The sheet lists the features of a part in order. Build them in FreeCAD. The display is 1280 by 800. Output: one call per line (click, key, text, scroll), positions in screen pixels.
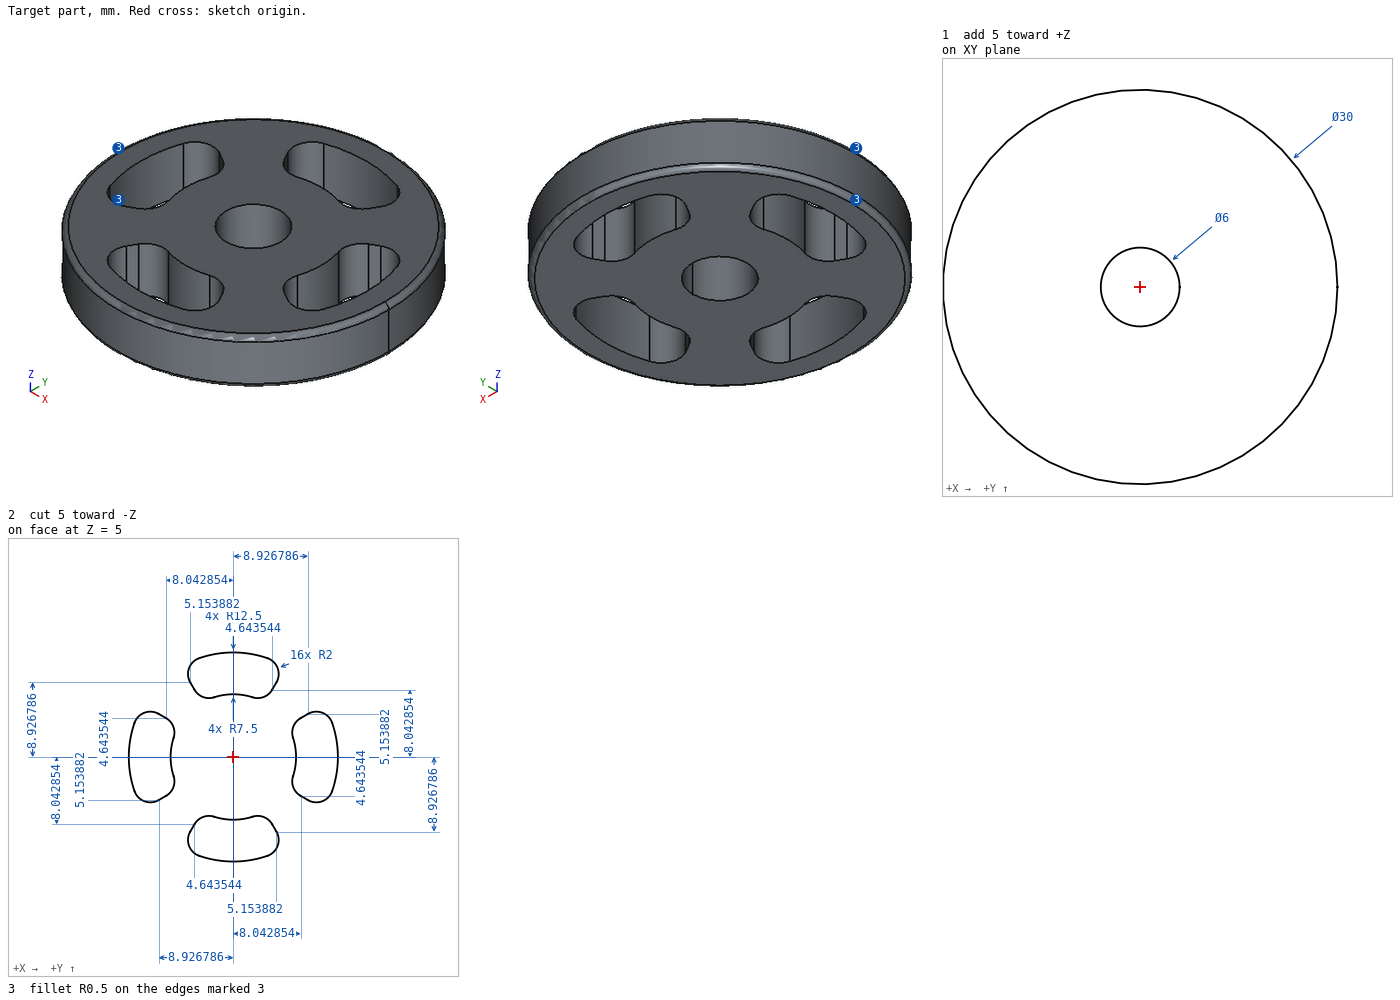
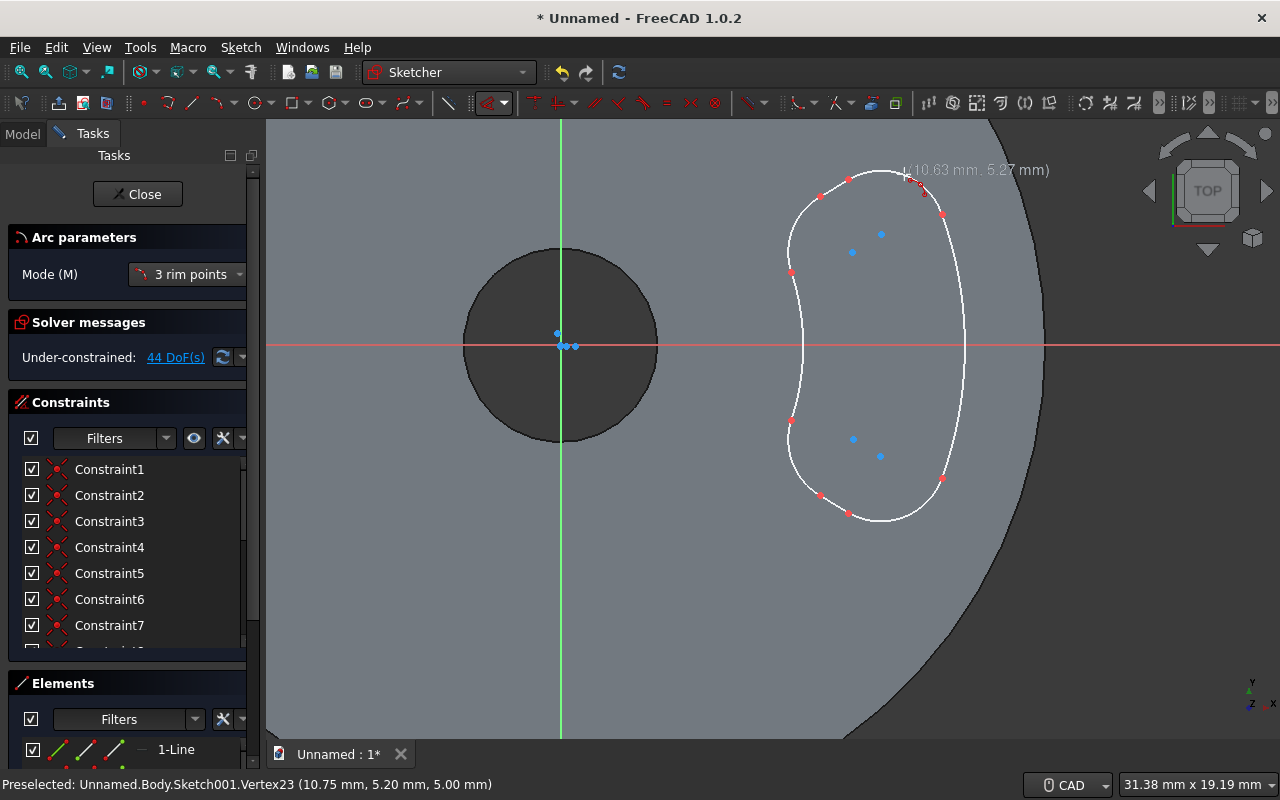
click(192, 104)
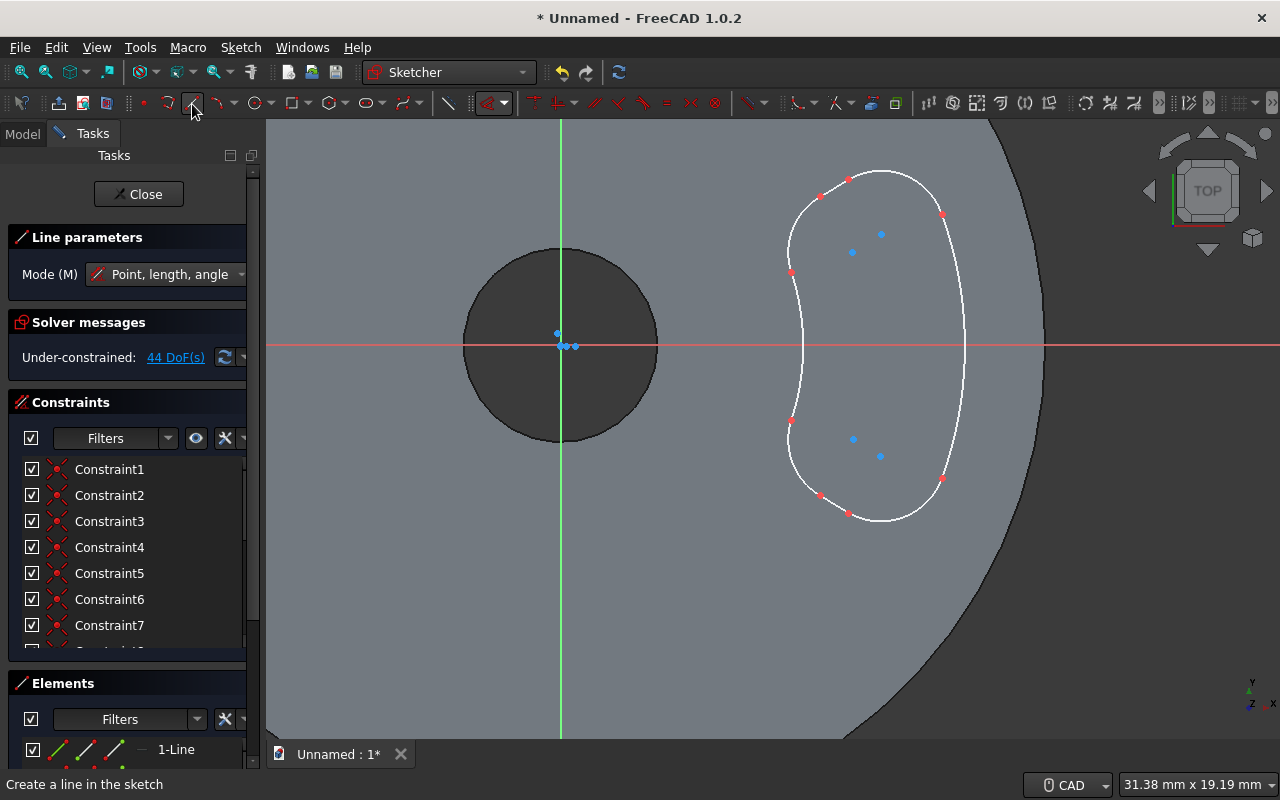
click(727, 634)
click(711, 605)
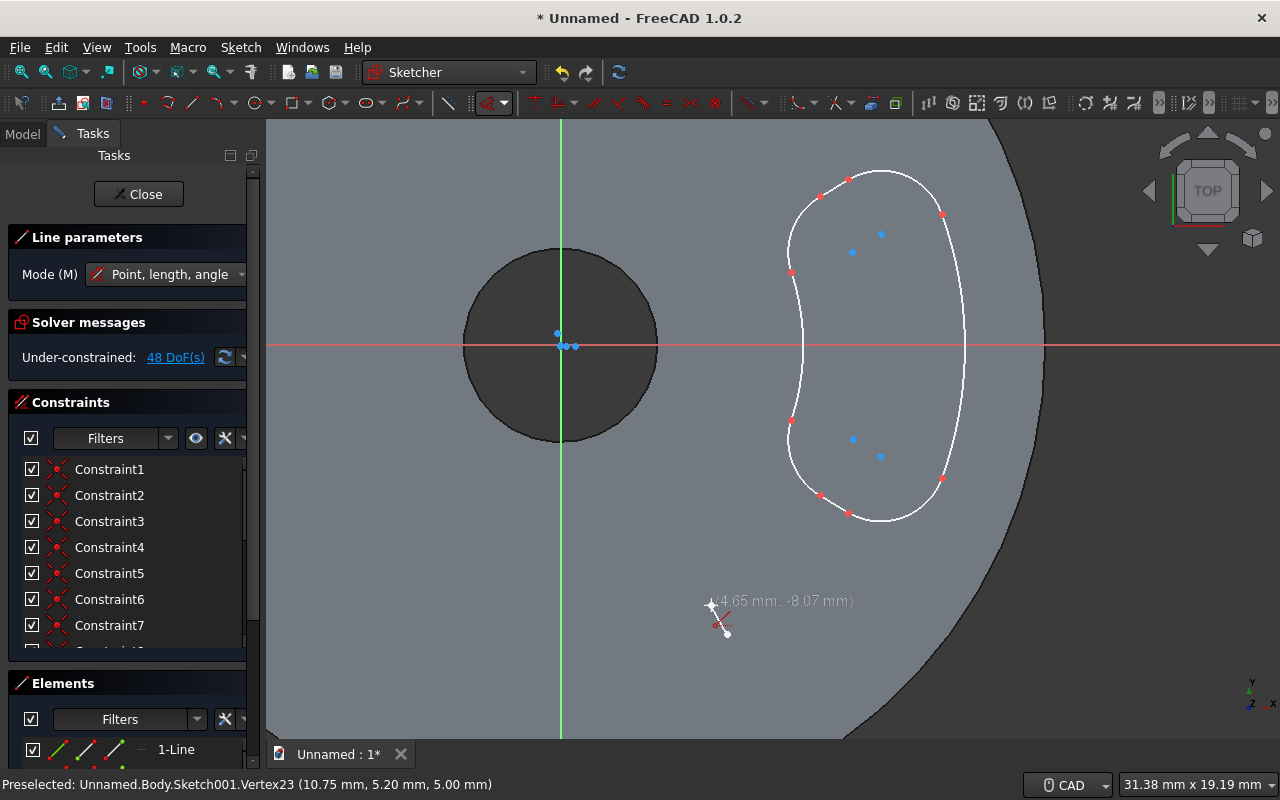
click(411, 605)
click(394, 634)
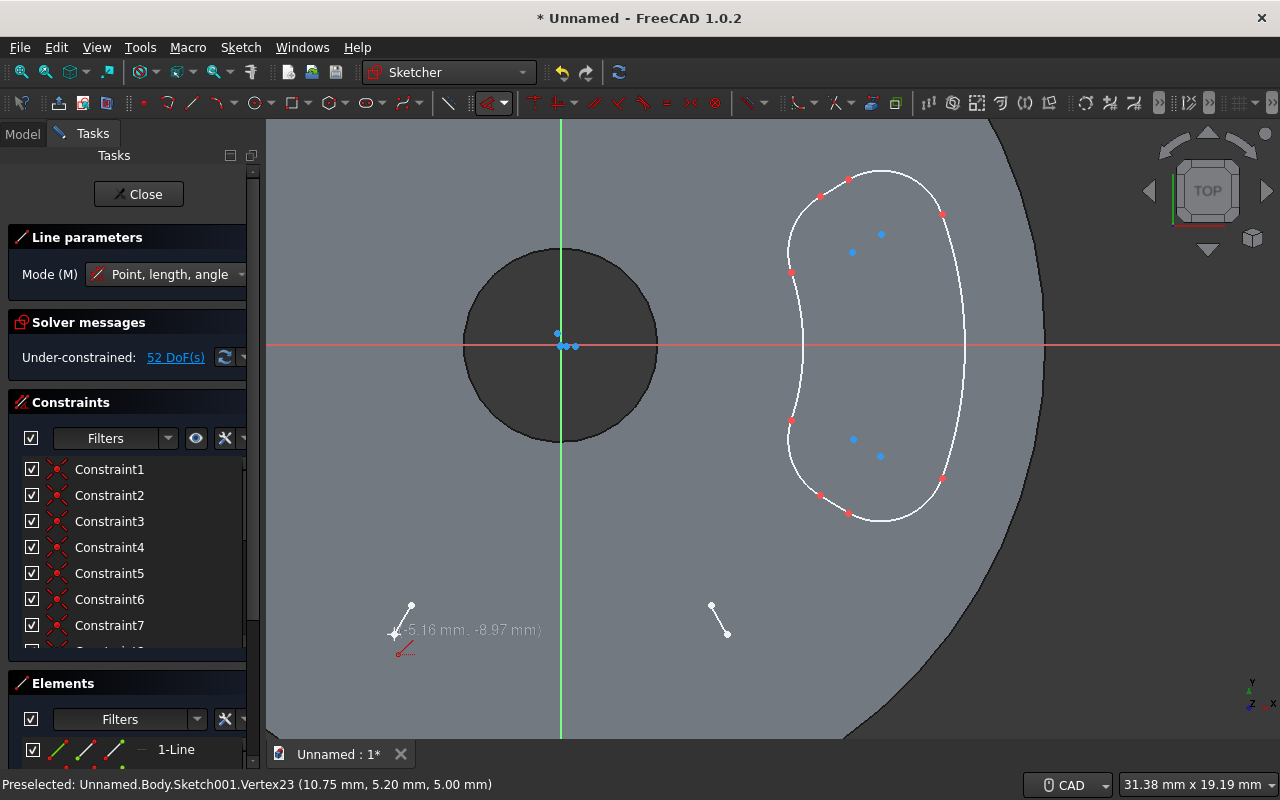
click(218, 104)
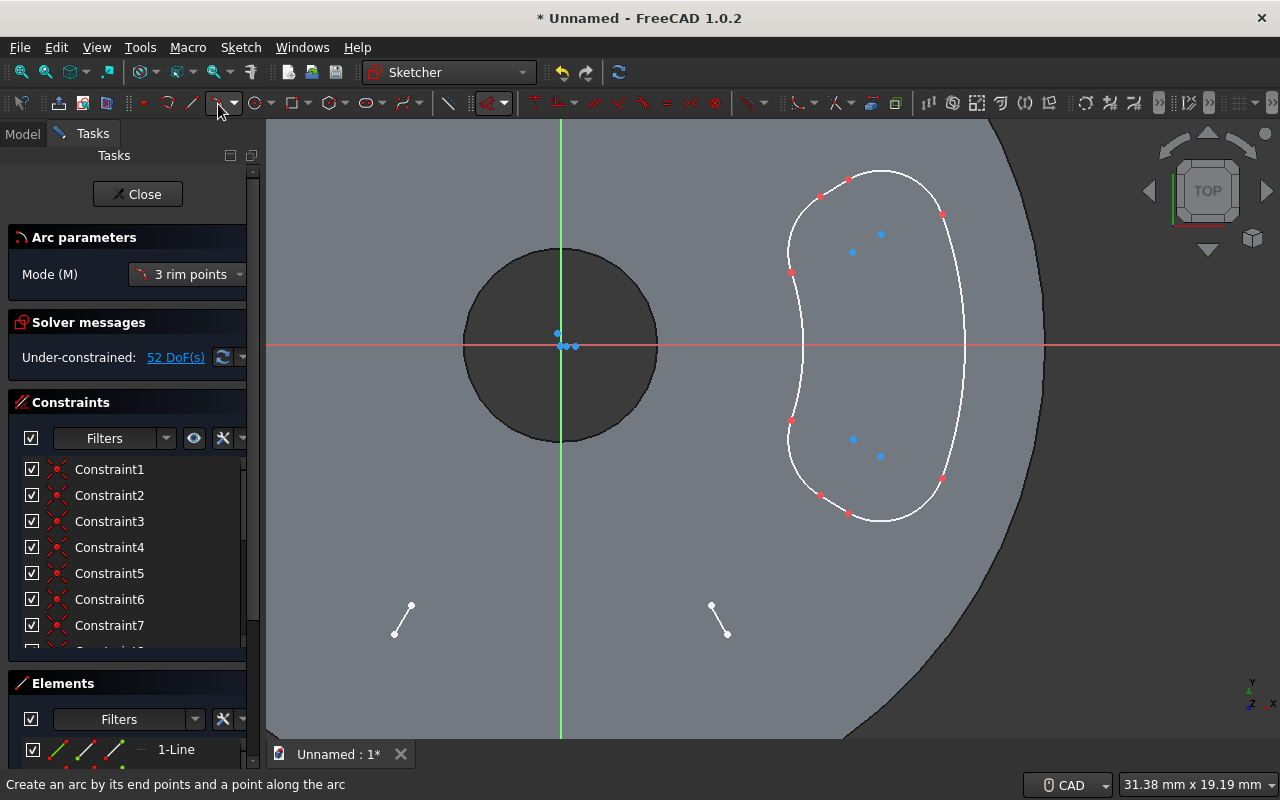
click(711, 606)
click(635, 576)
click(678, 577)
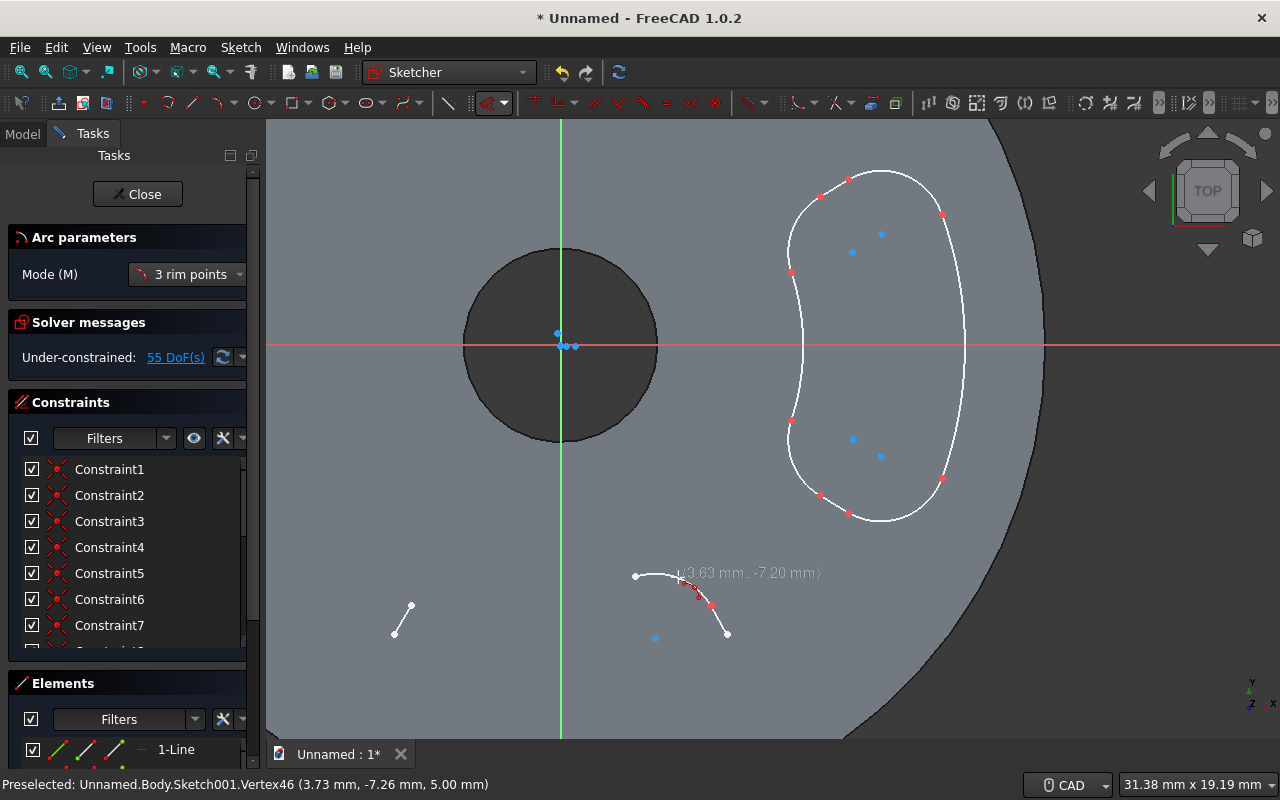
click(635, 577)
click(486, 576)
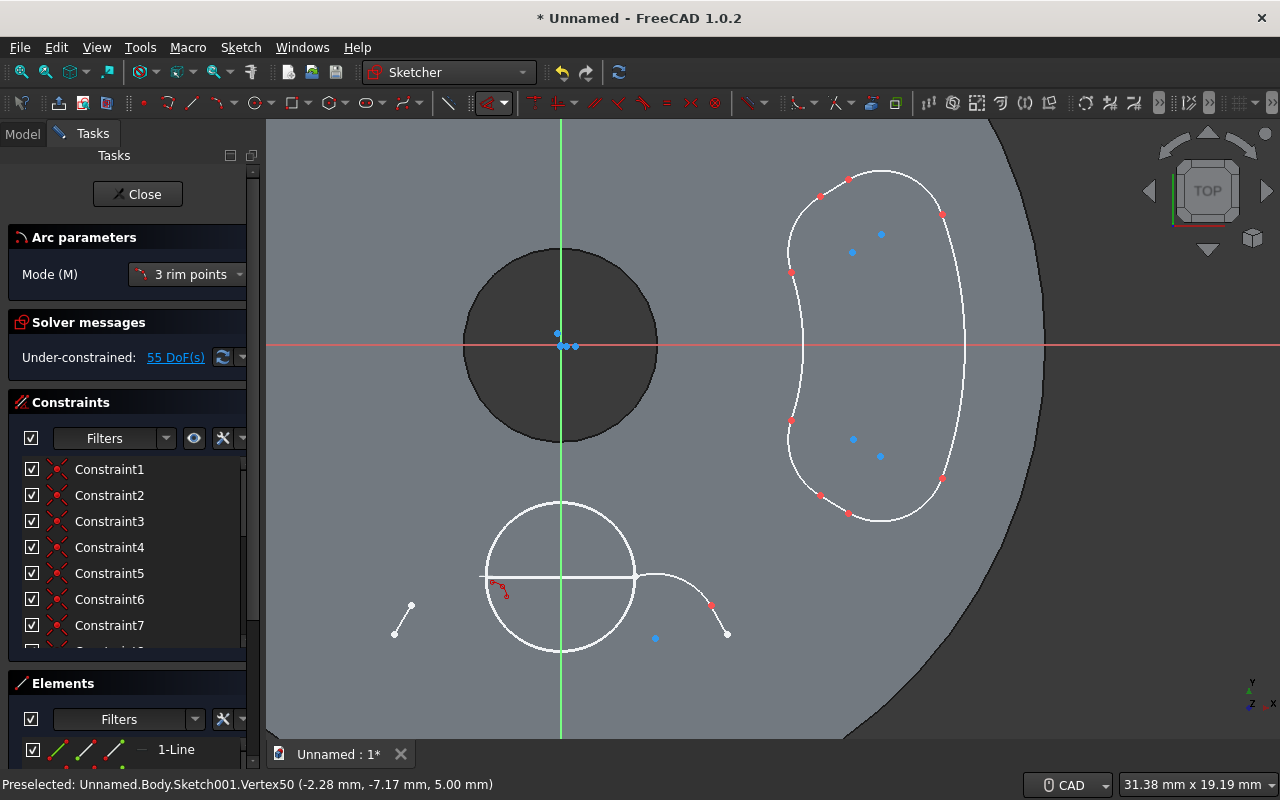
scroll(546, 587, up, 2)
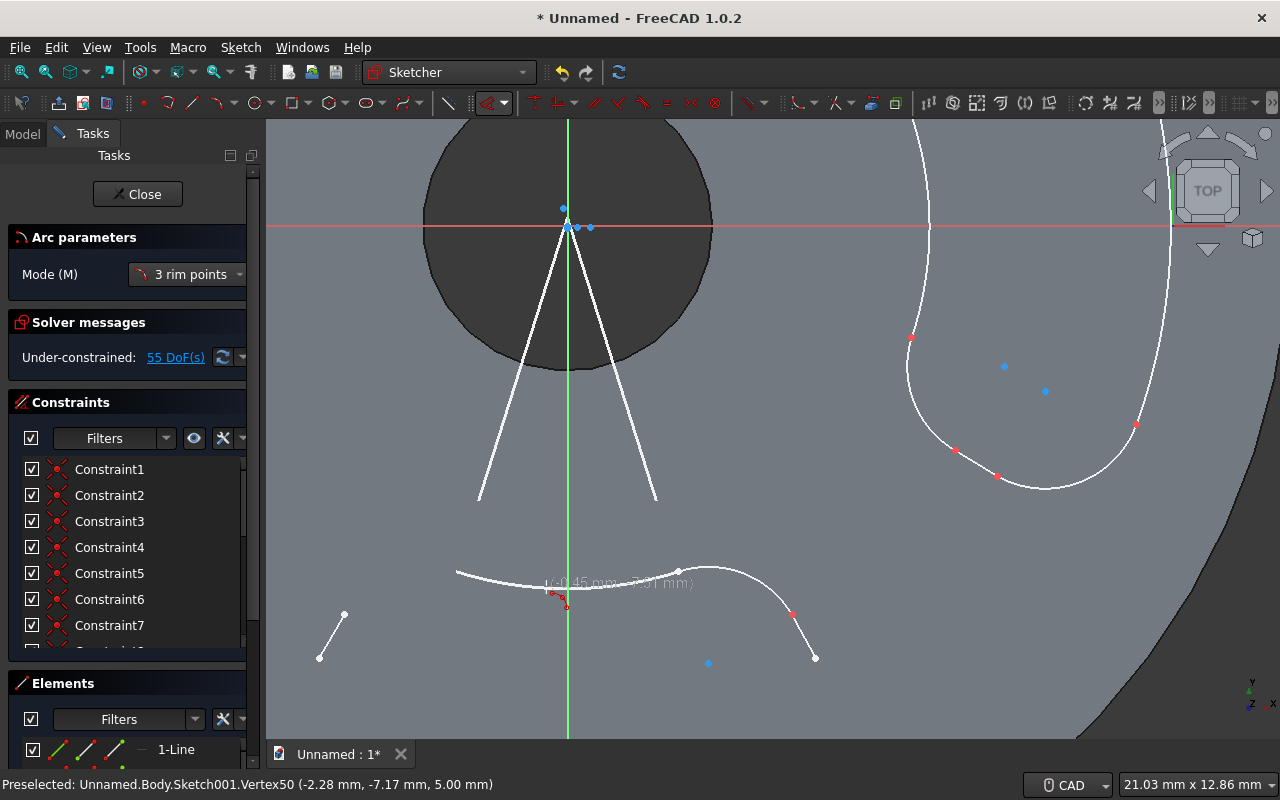
click(545, 587)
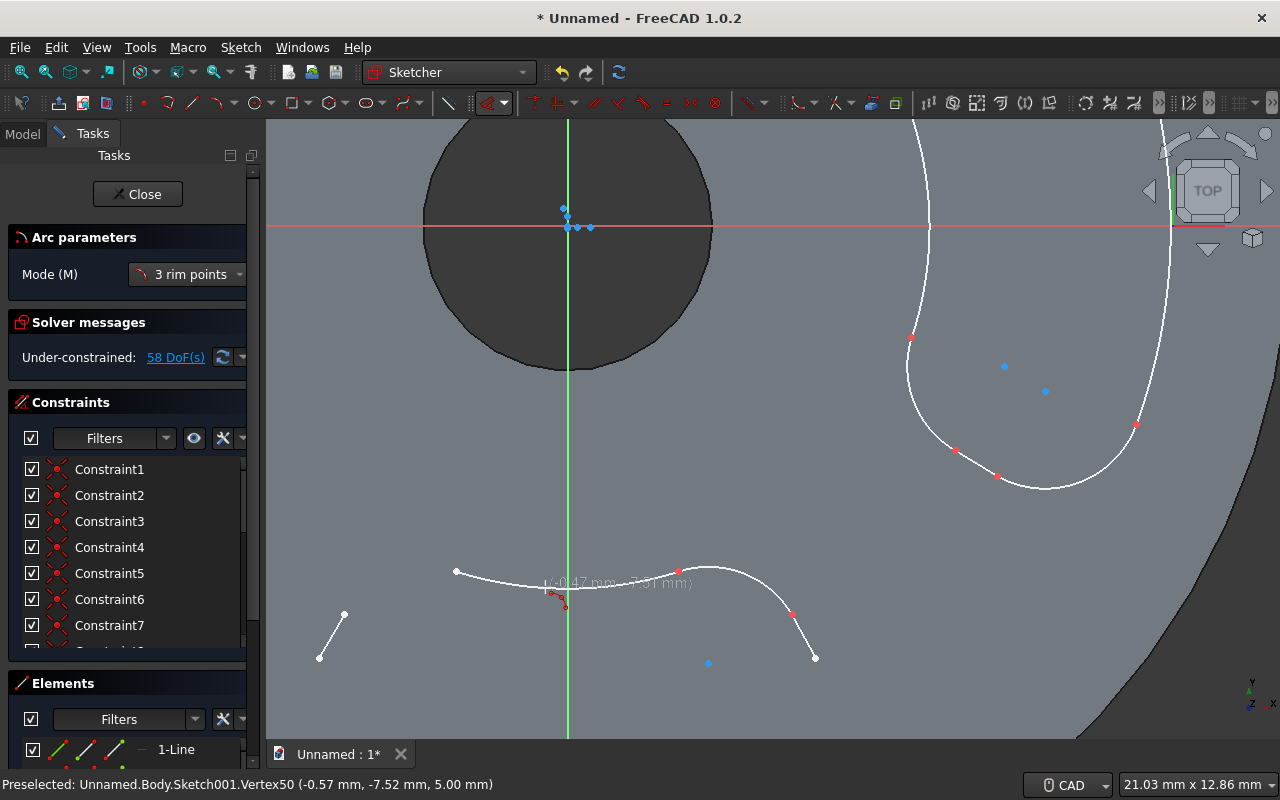
click(456, 572)
click(344, 615)
click(393, 572)